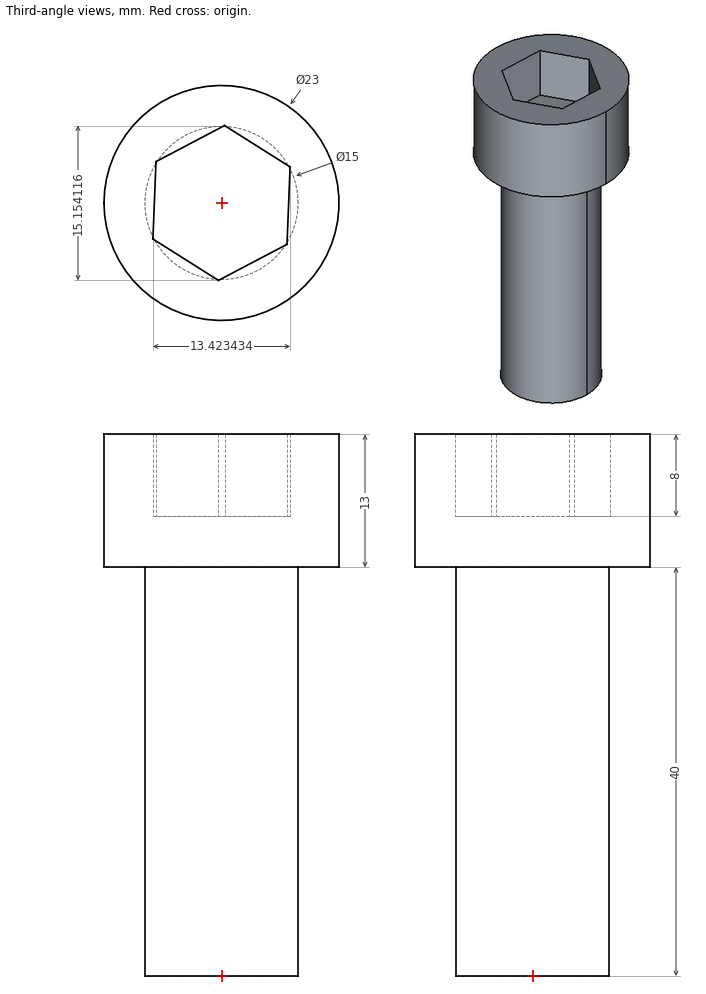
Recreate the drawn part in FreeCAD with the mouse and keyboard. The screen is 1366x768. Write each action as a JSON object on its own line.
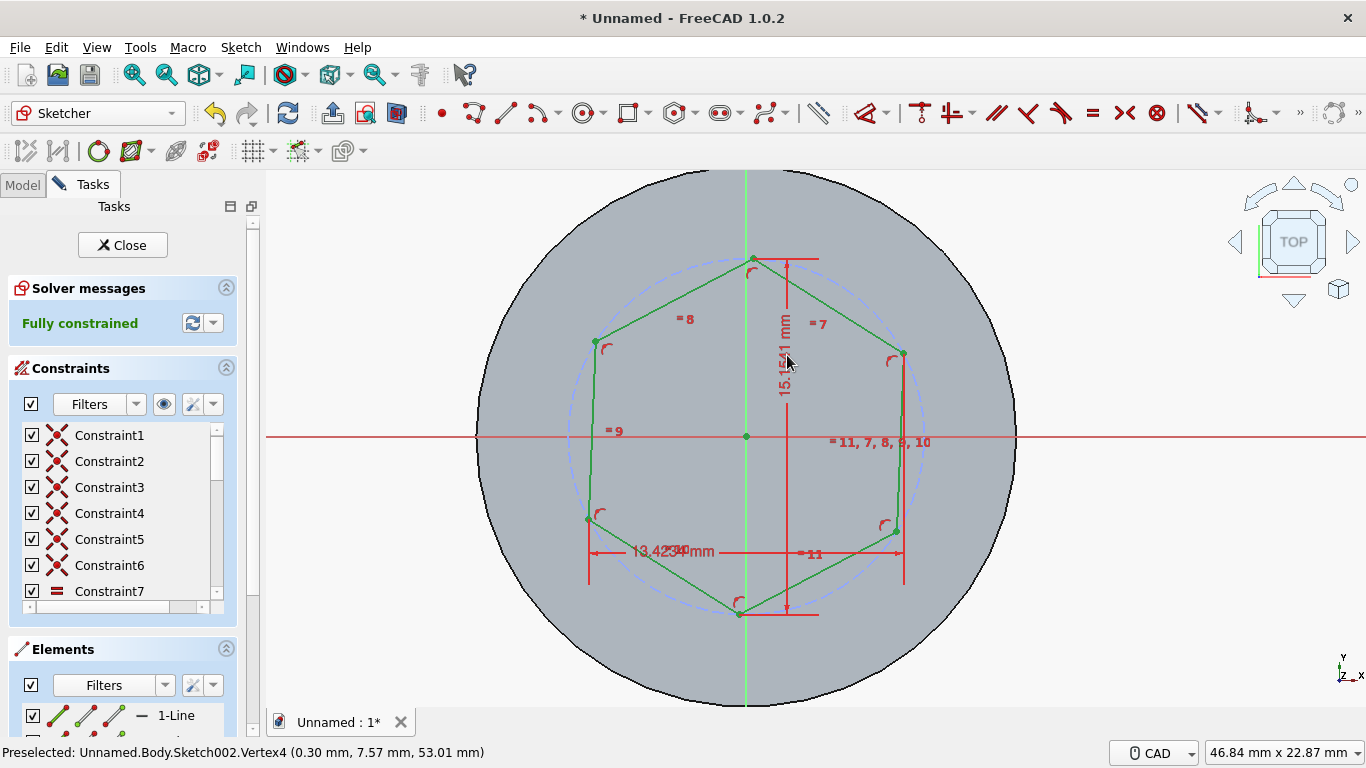
{"action": "left_click", "coordinate": [123, 245]}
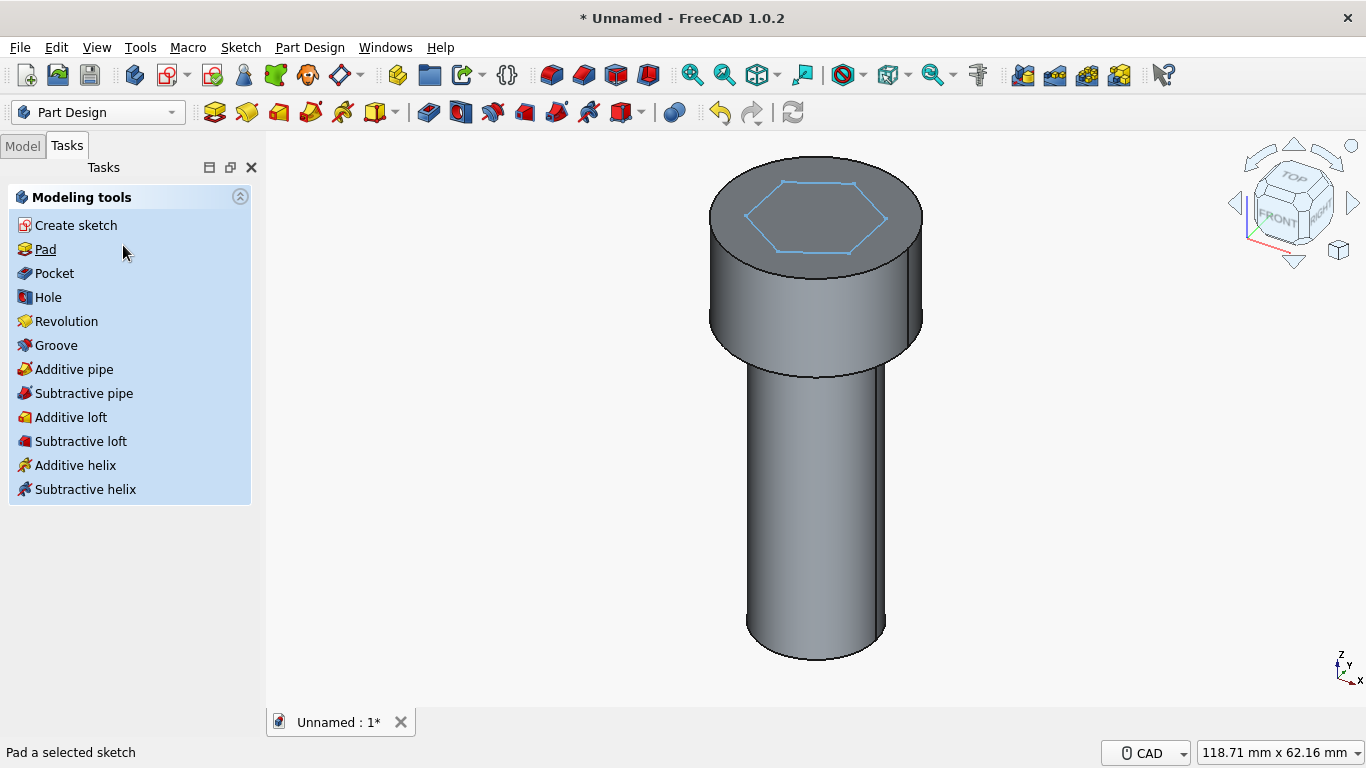
{"action": "left_click", "coordinate": [430, 112]}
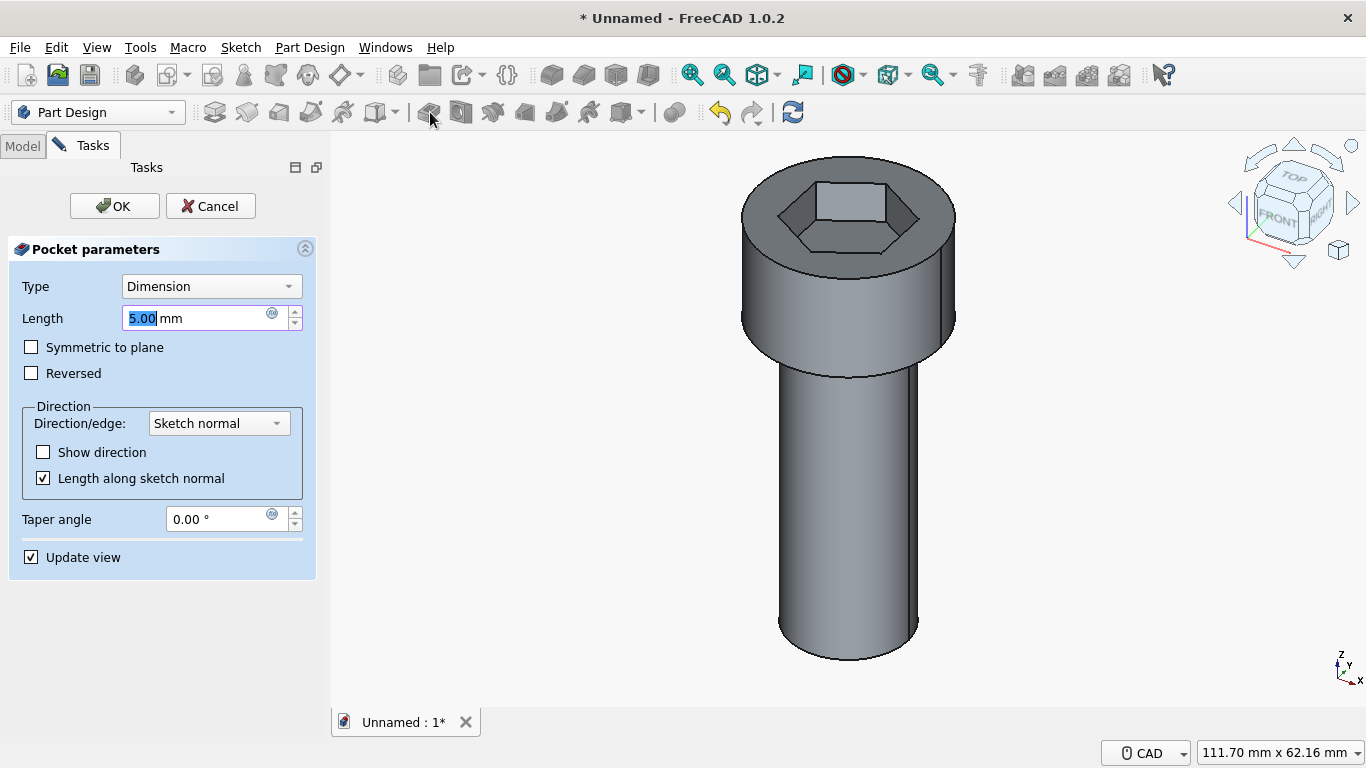
{"action": "type", "text": "8"}
{"action": "key", "text": "Tab"}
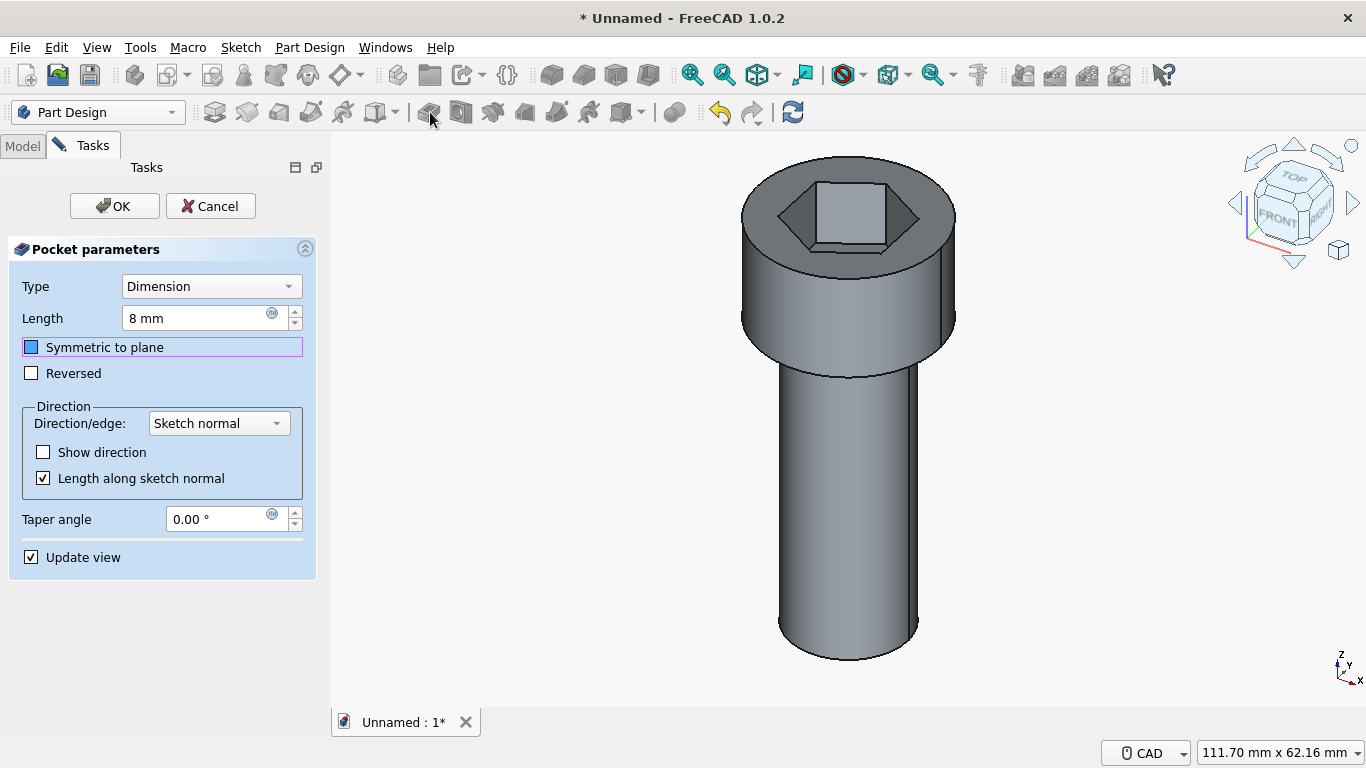
{"action": "left_click", "coordinate": [115, 206]}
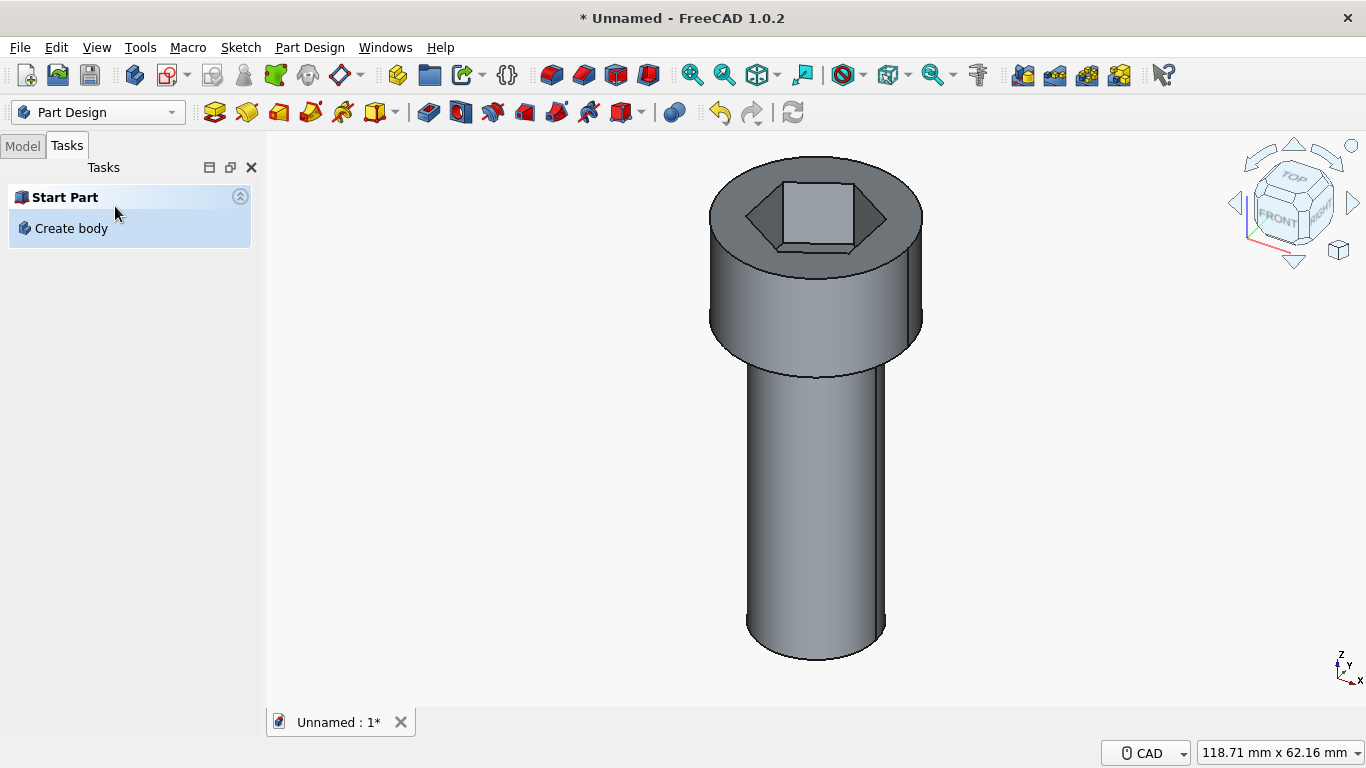
{"action": "key", "text": "0"}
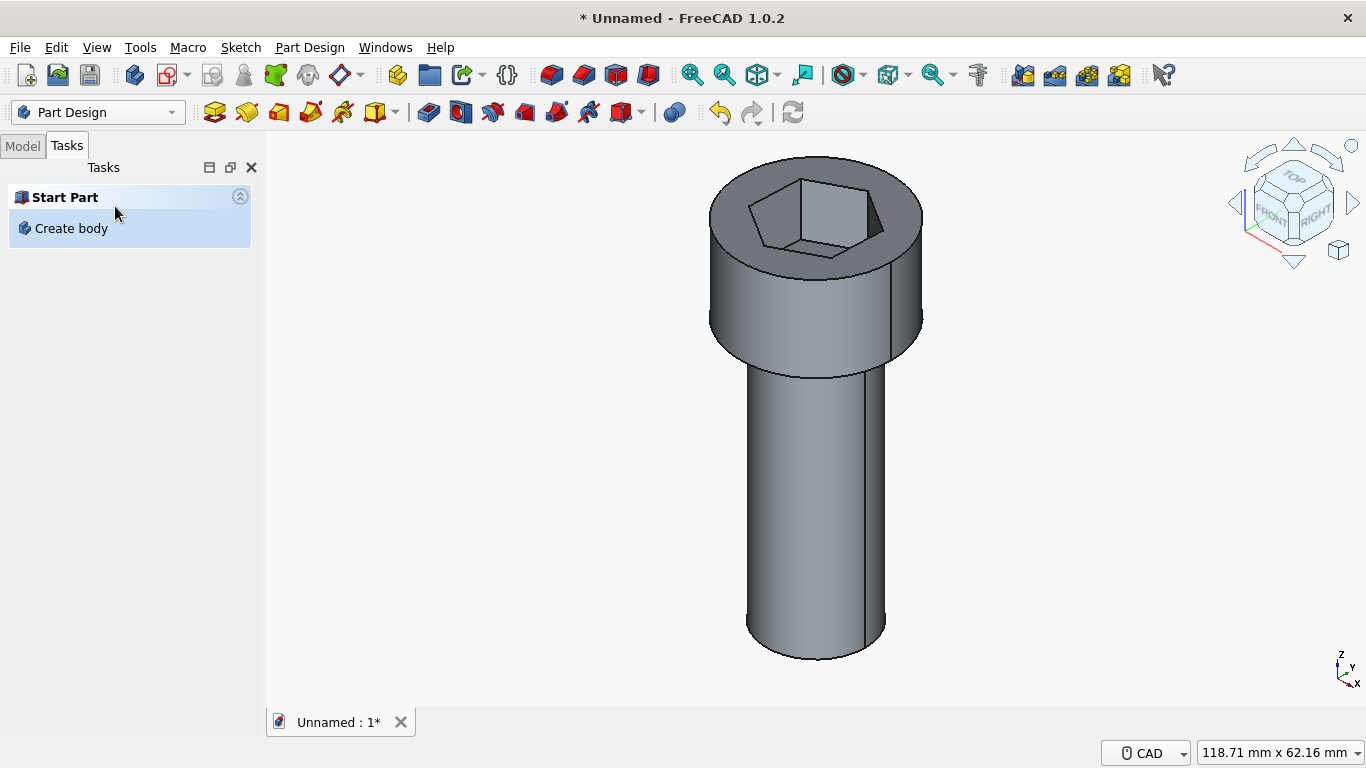
{"action": "left_click", "coordinate": [694, 76]}